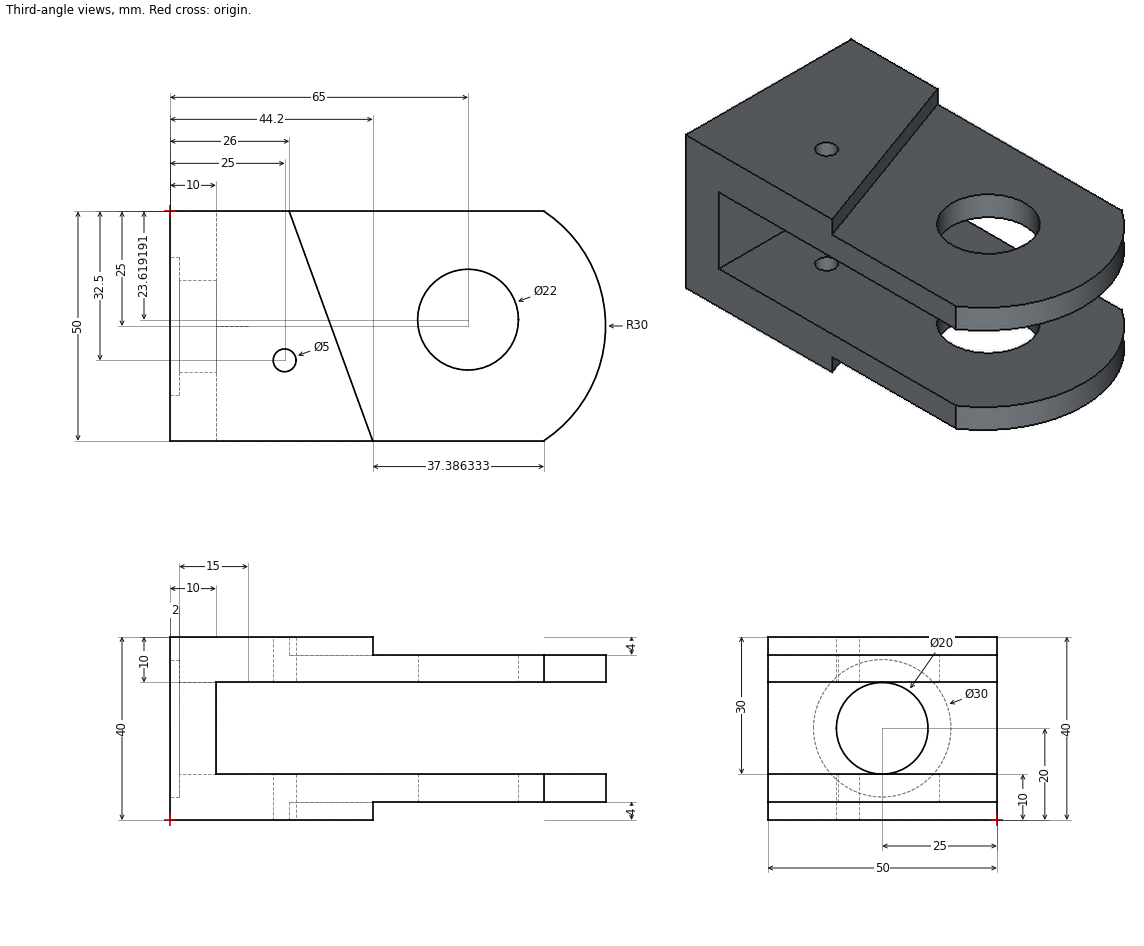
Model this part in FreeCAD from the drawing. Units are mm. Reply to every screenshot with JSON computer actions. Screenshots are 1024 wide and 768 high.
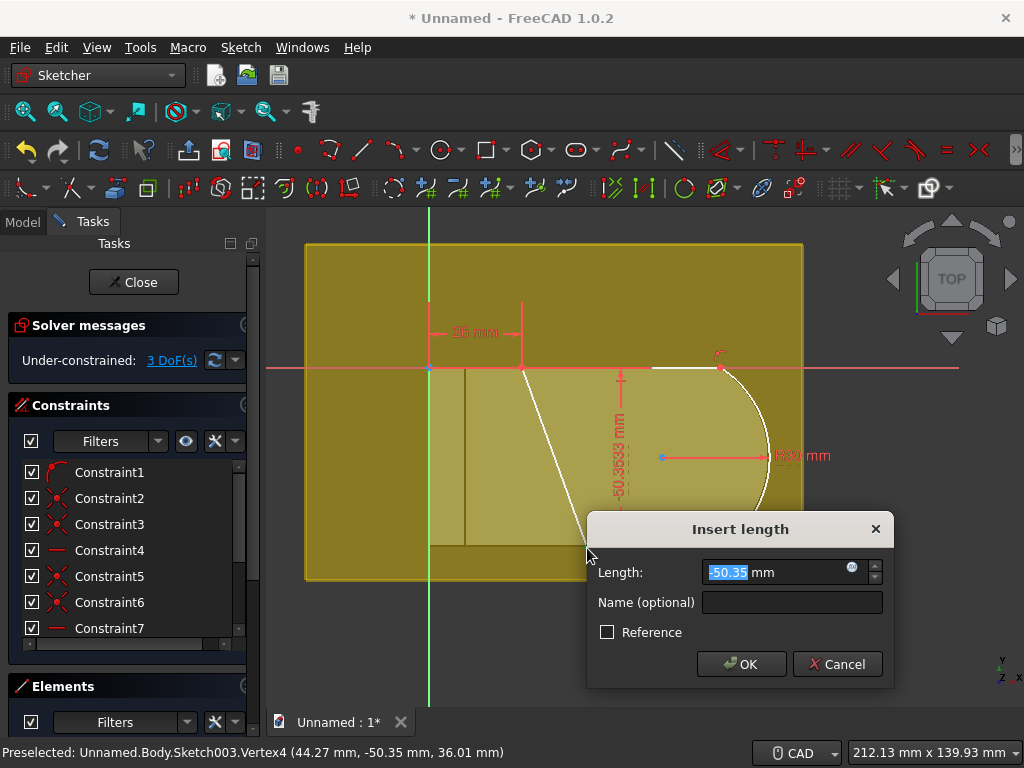
{"action": "type", "text": "-50"}
{"action": "key", "text": "Return"}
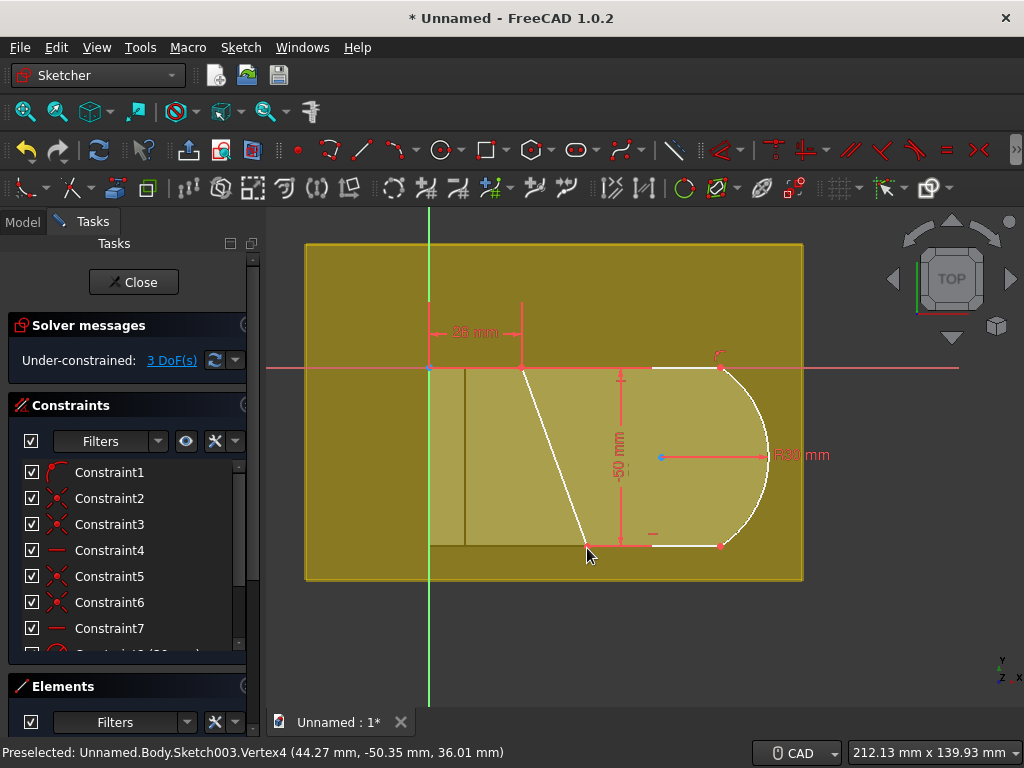
{"action": "left_click", "coordinate": [661, 457]}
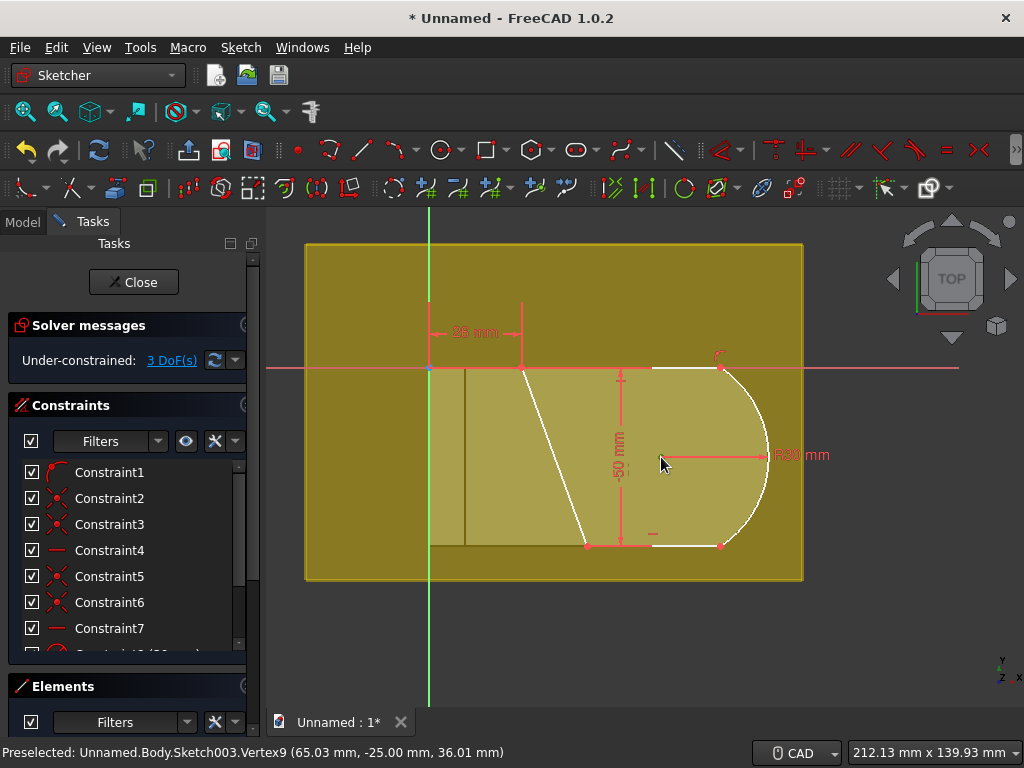
{"action": "key", "text": "l"}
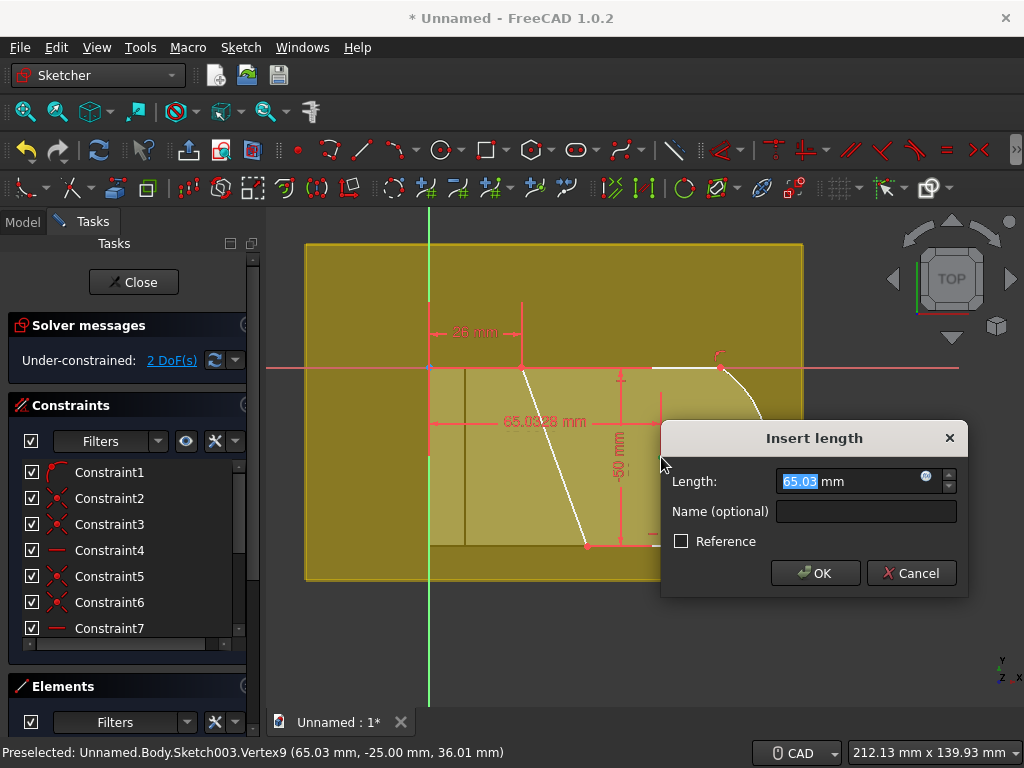
{"action": "type", "text": "65"}
{"action": "key", "text": "Return"}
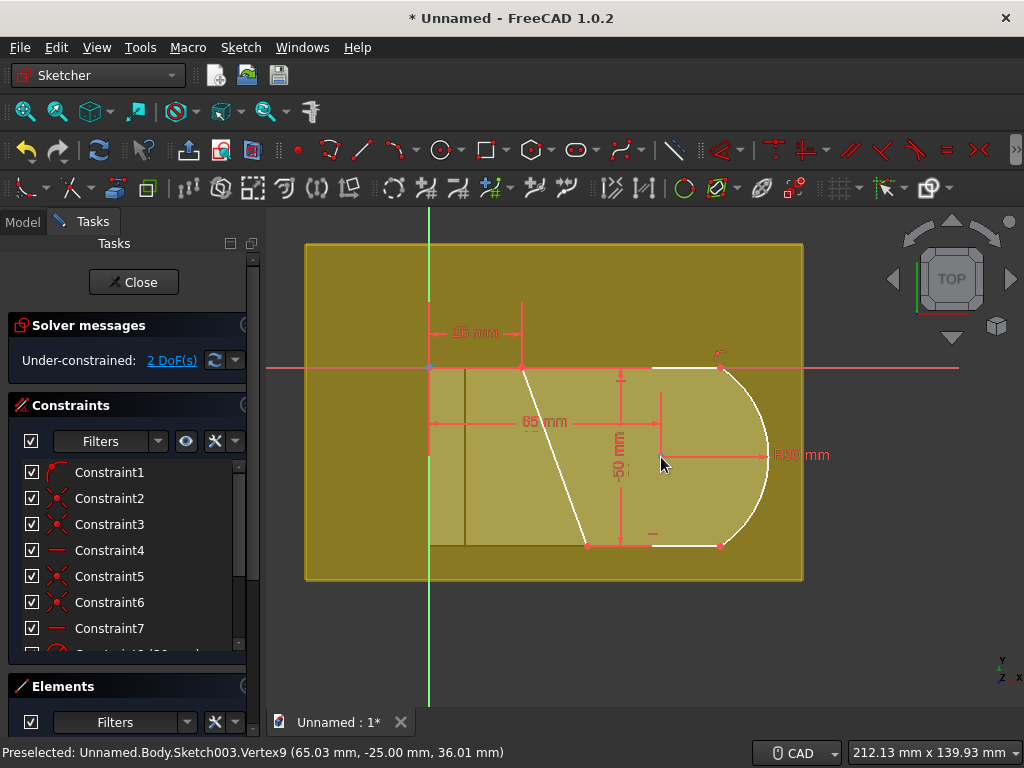
{"action": "left_click", "coordinate": [661, 457]}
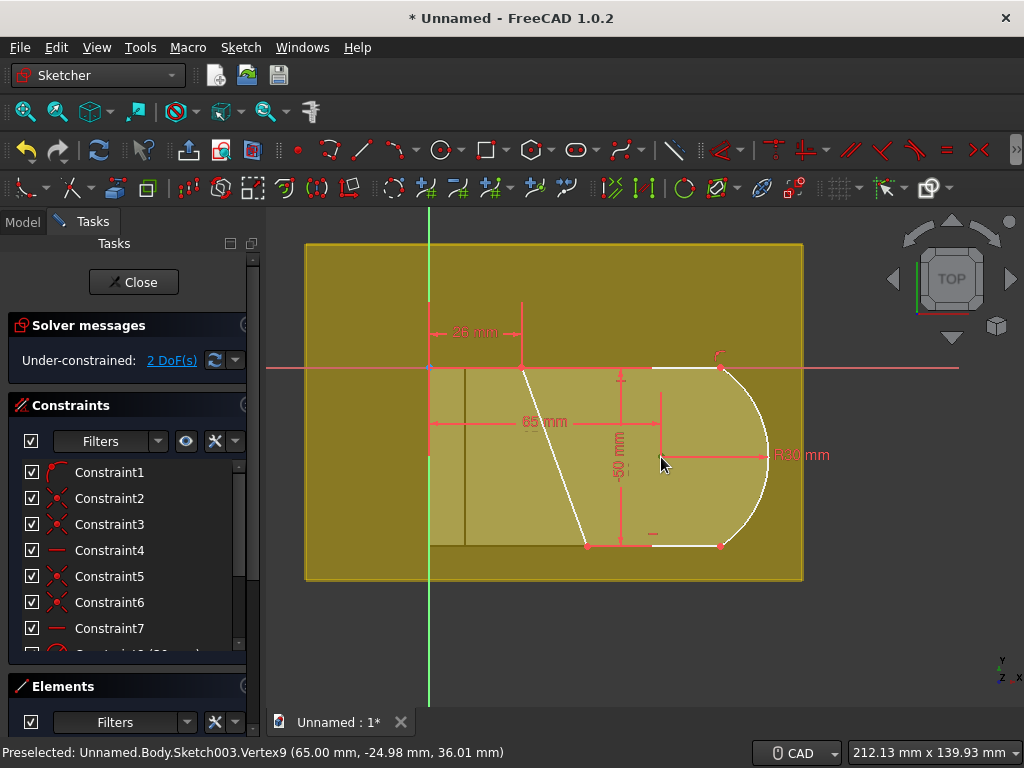
{"action": "key", "text": "i"}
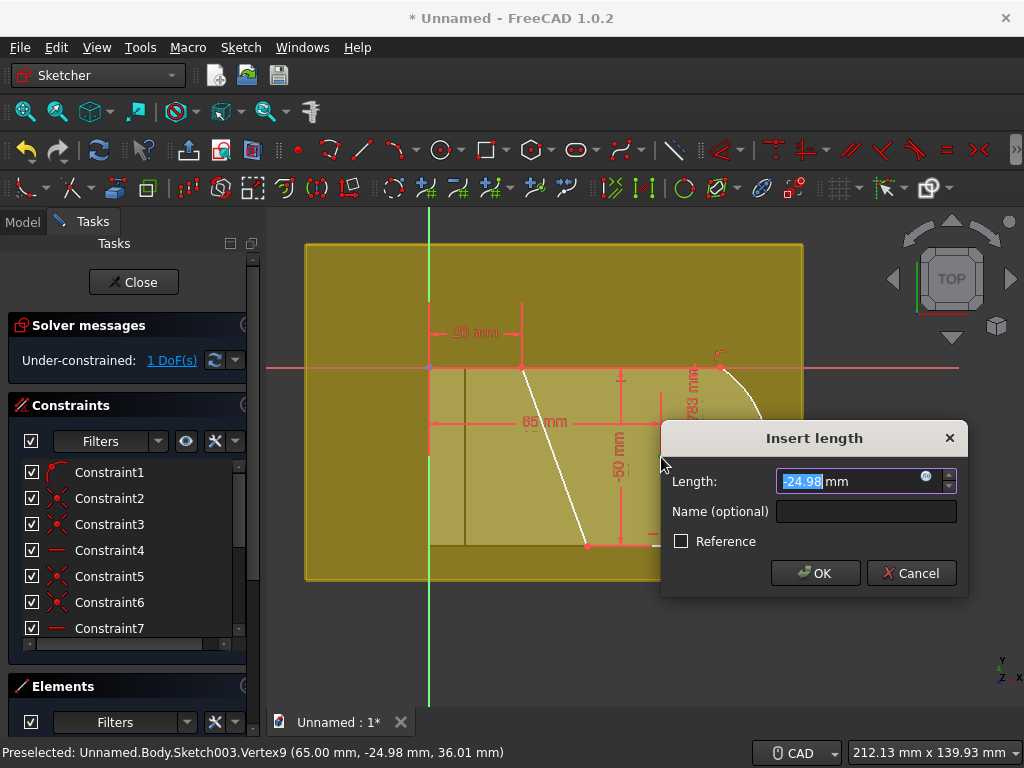
{"action": "type", "text": "-25"}
{"action": "key", "text": "Return"}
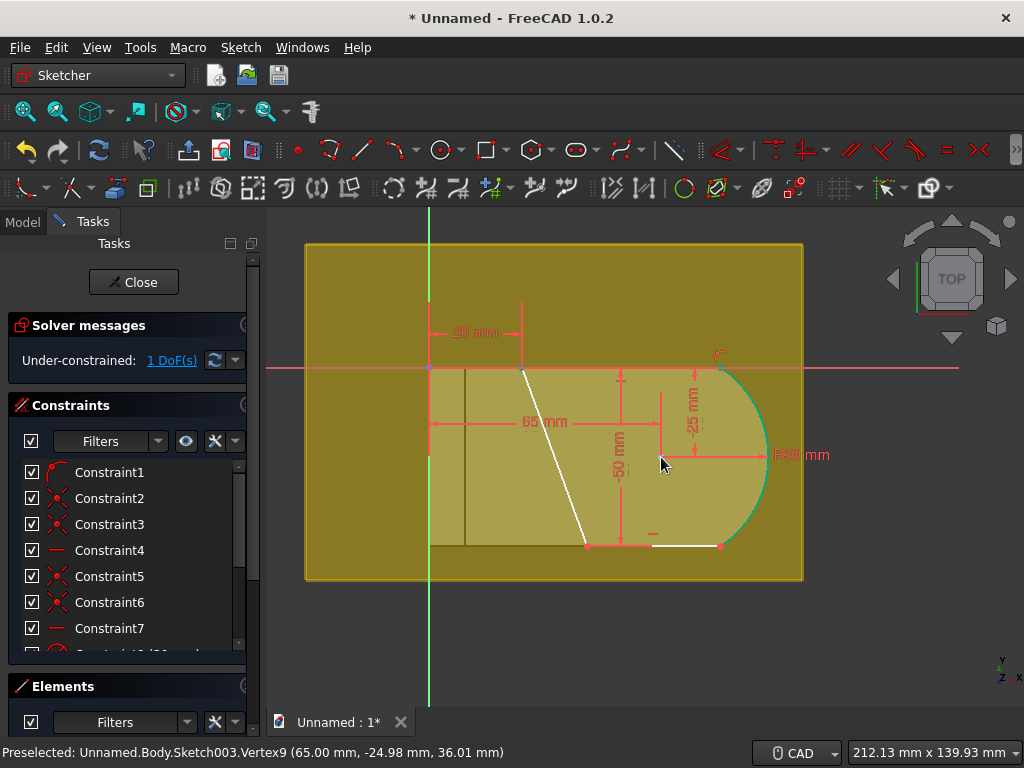
{"action": "left_click", "coordinate": [627, 546]}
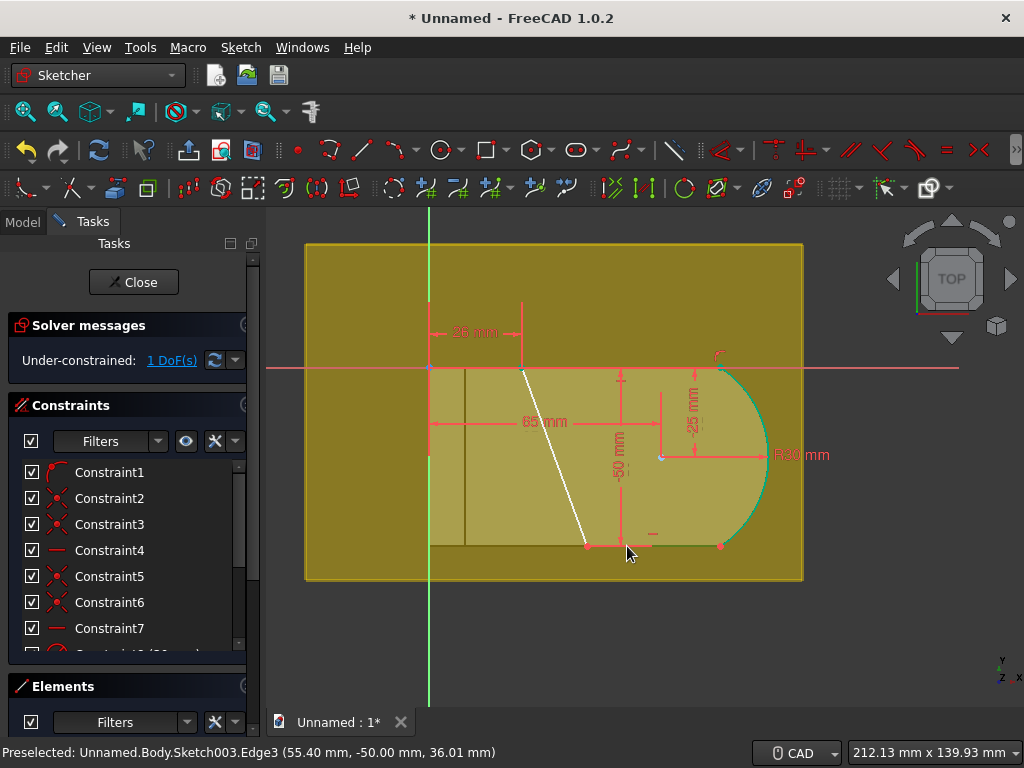
{"action": "key", "text": "l"}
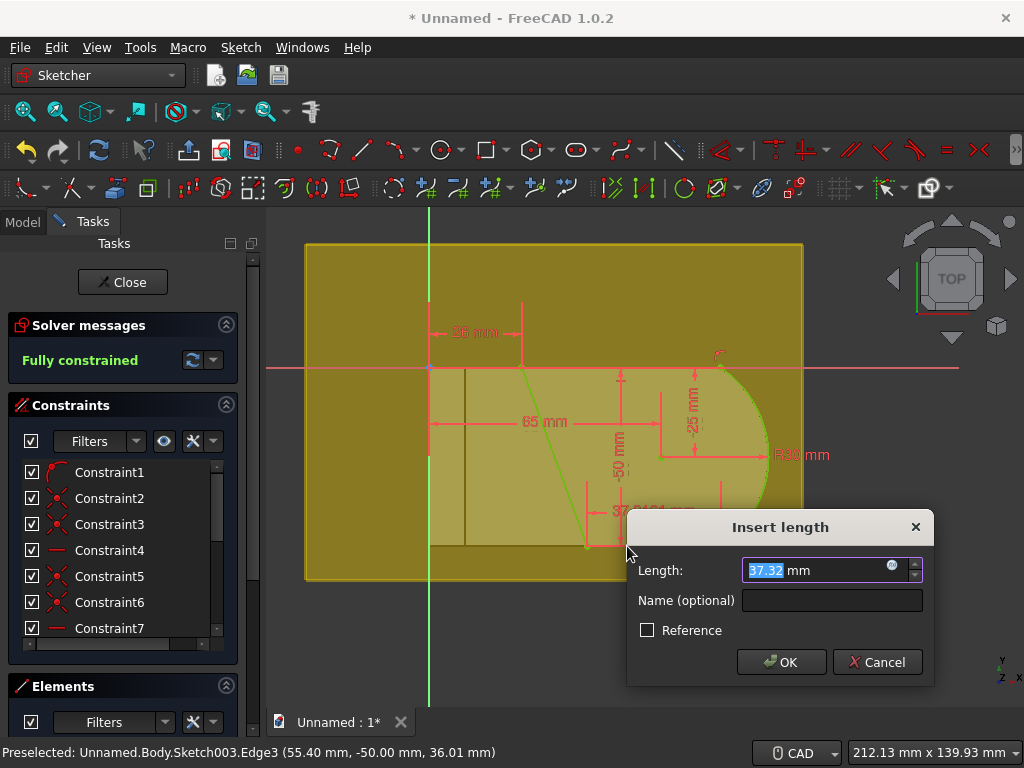
{"action": "type", "text": "37.386333"}
{"action": "key", "text": "Return"}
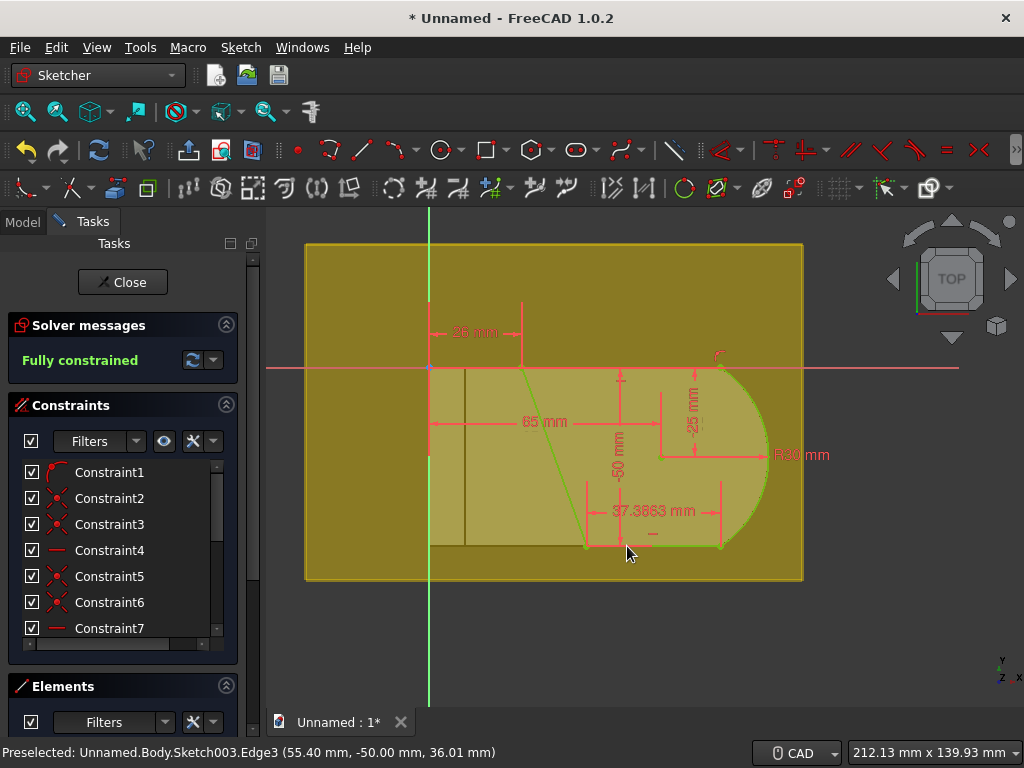
{"action": "left_click", "coordinate": [123, 282]}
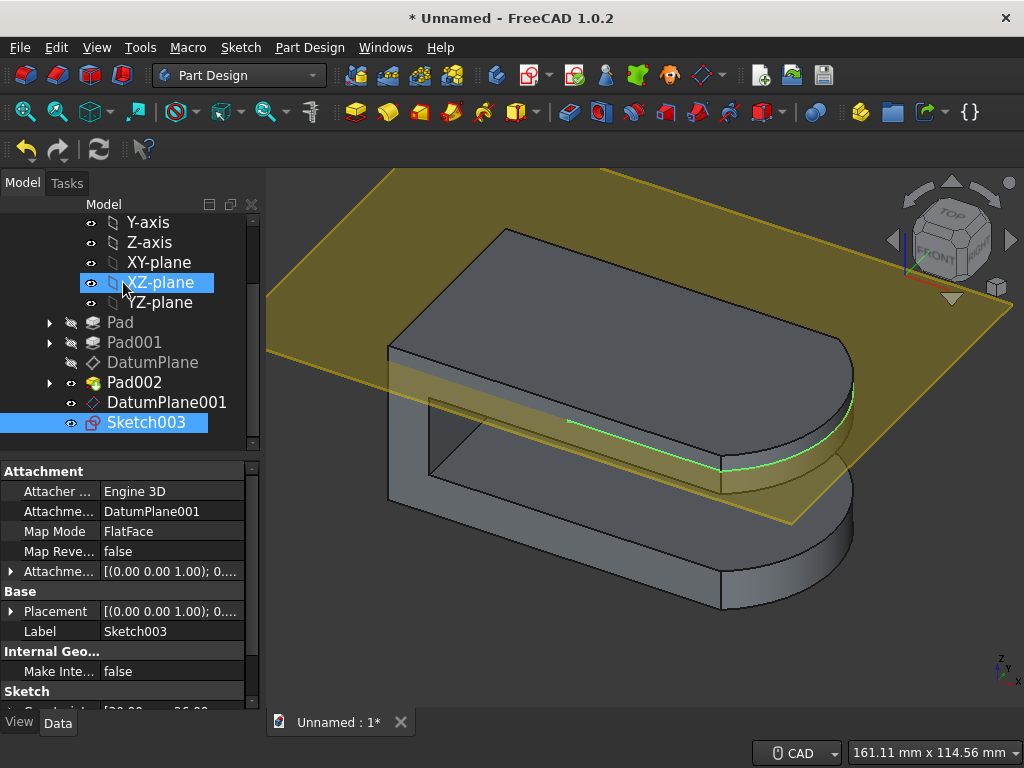
{"action": "left_click", "coordinate": [570, 112]}